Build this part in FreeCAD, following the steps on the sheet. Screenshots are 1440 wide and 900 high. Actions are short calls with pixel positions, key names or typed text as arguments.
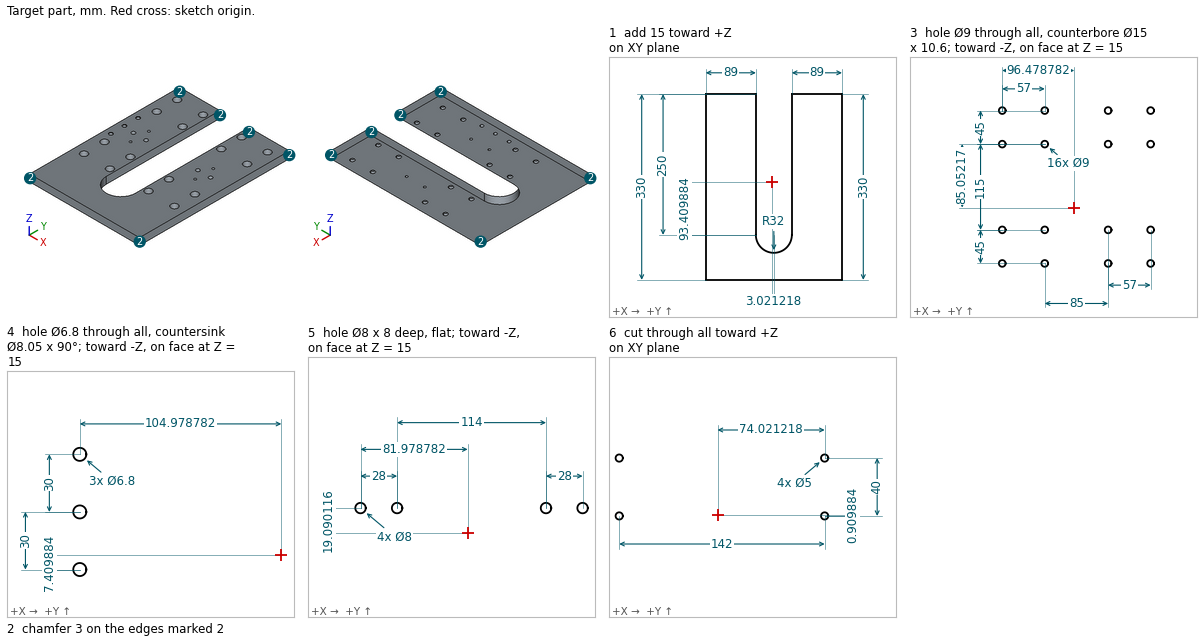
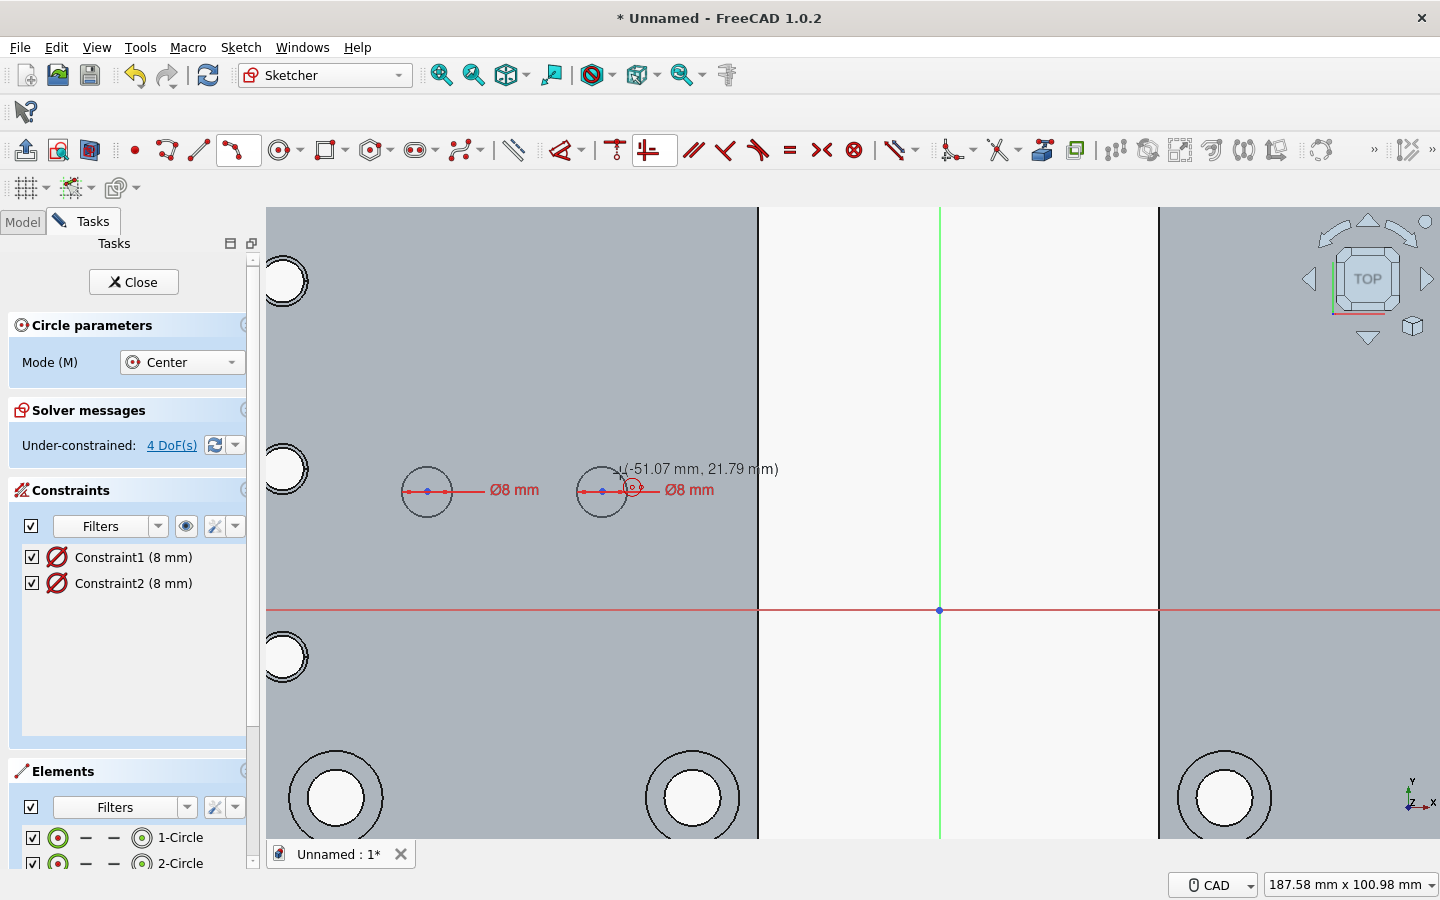
scroll(431, 492, down, 2)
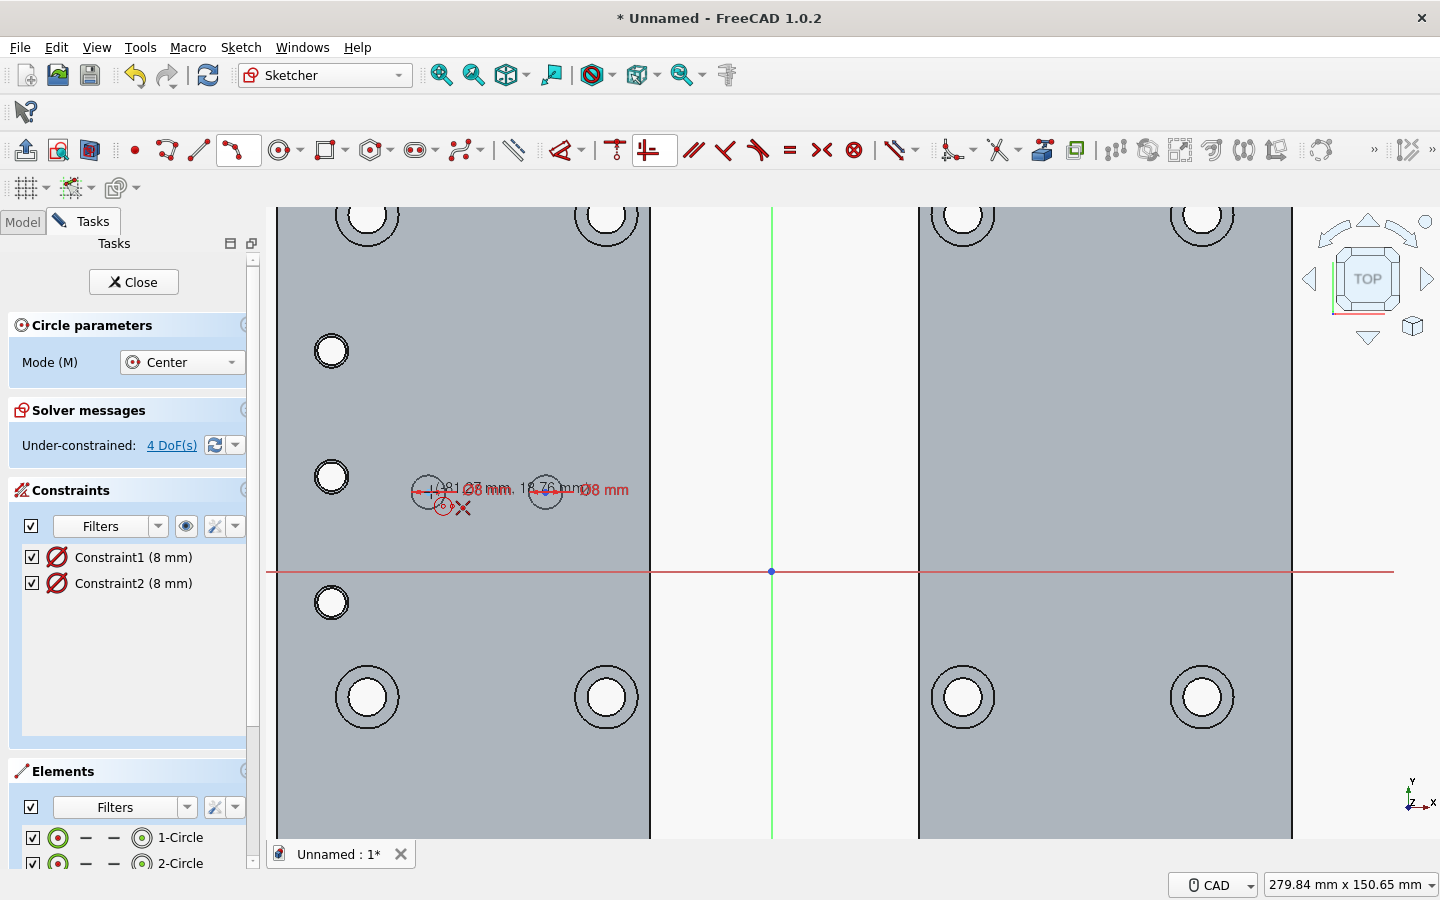
scroll(1024, 491, up, 2)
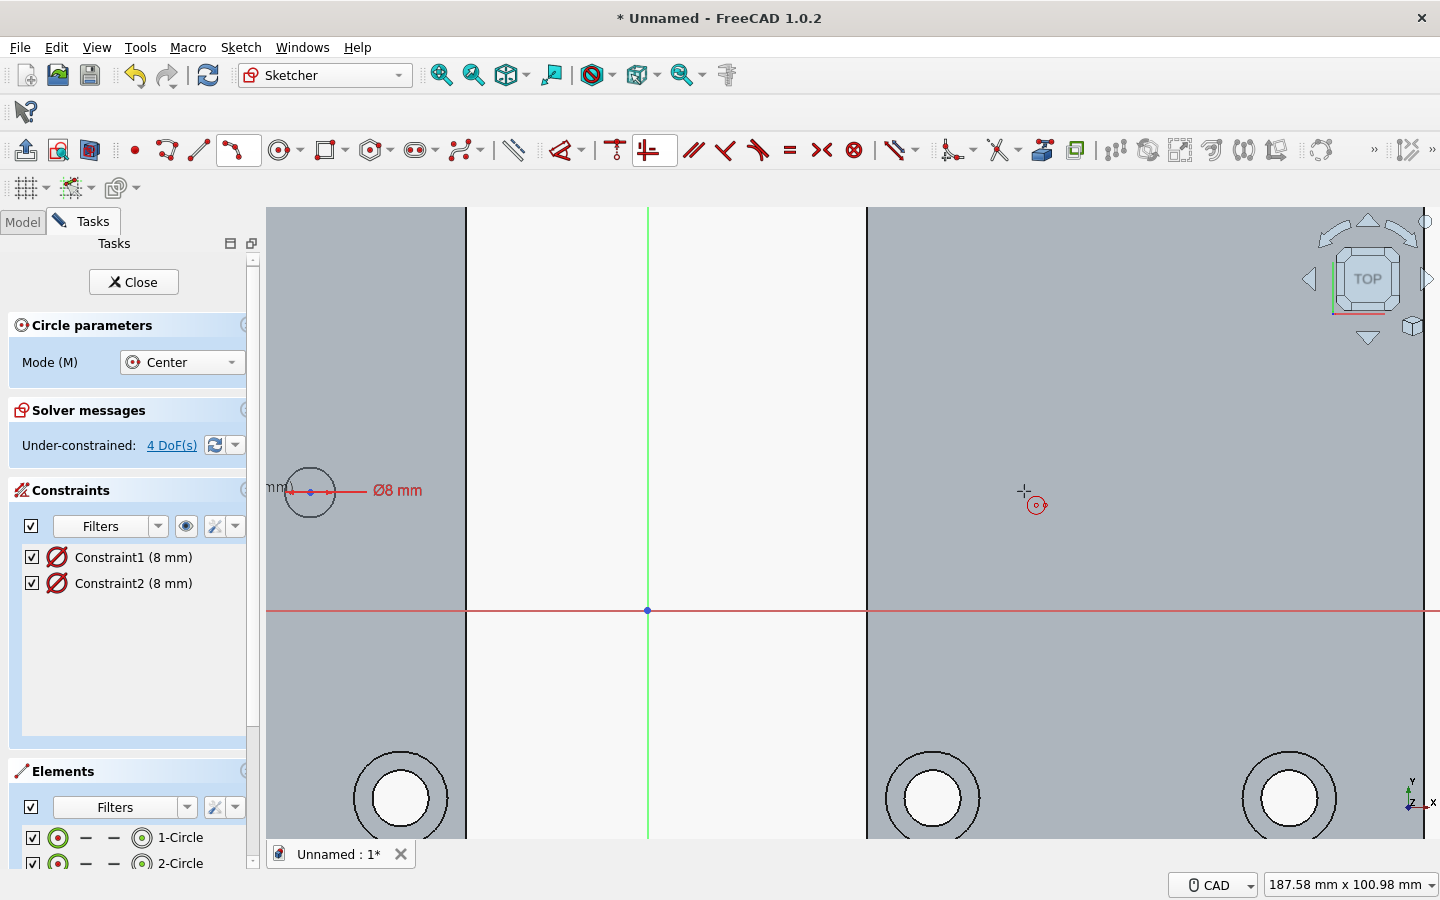
click(1023, 491)
move(1041, 474)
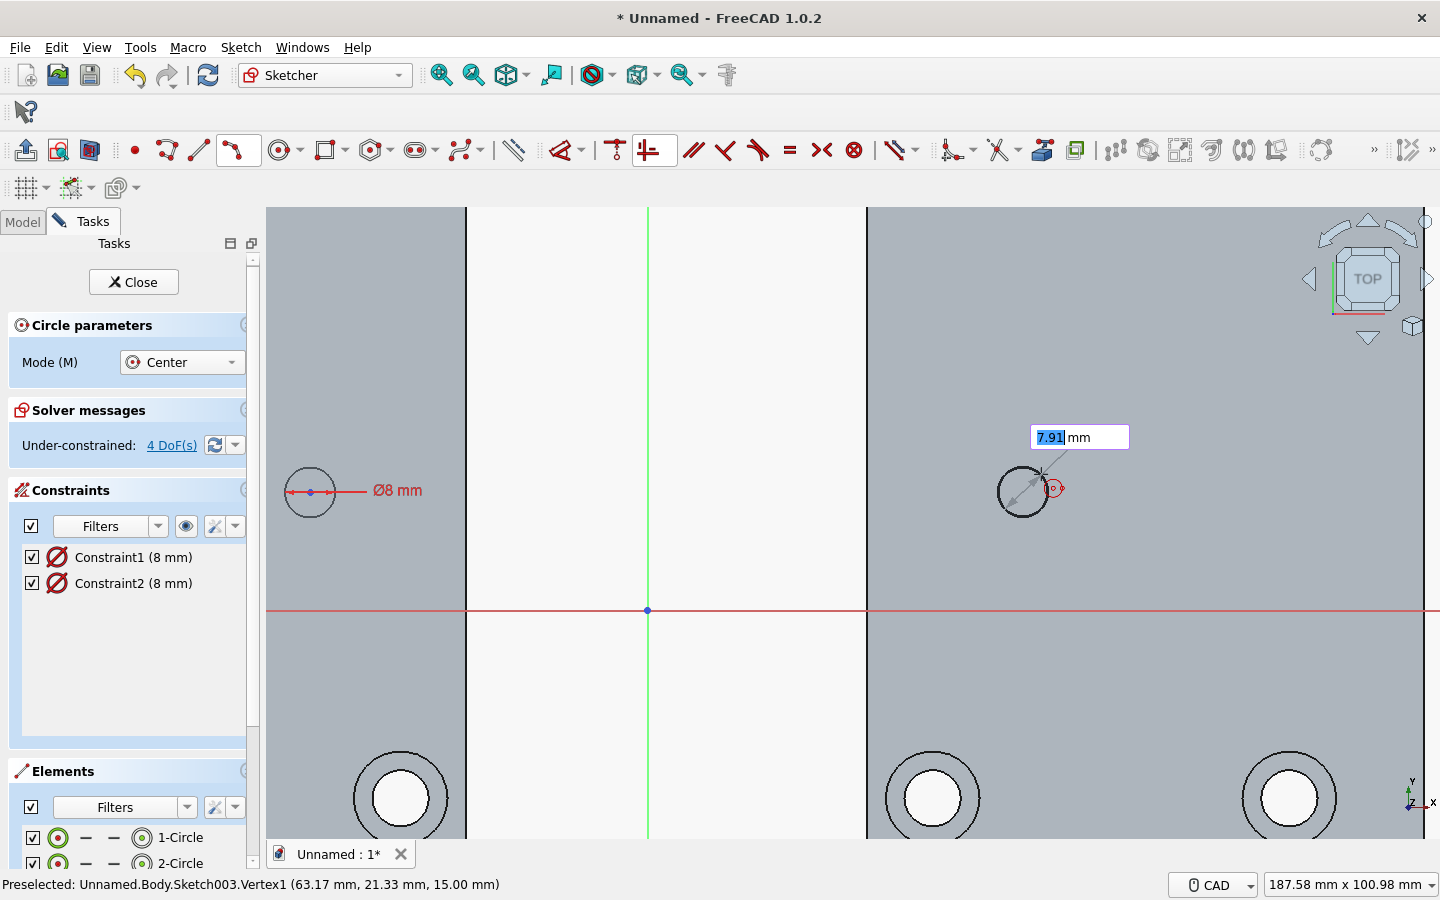
text(8)
key(Return)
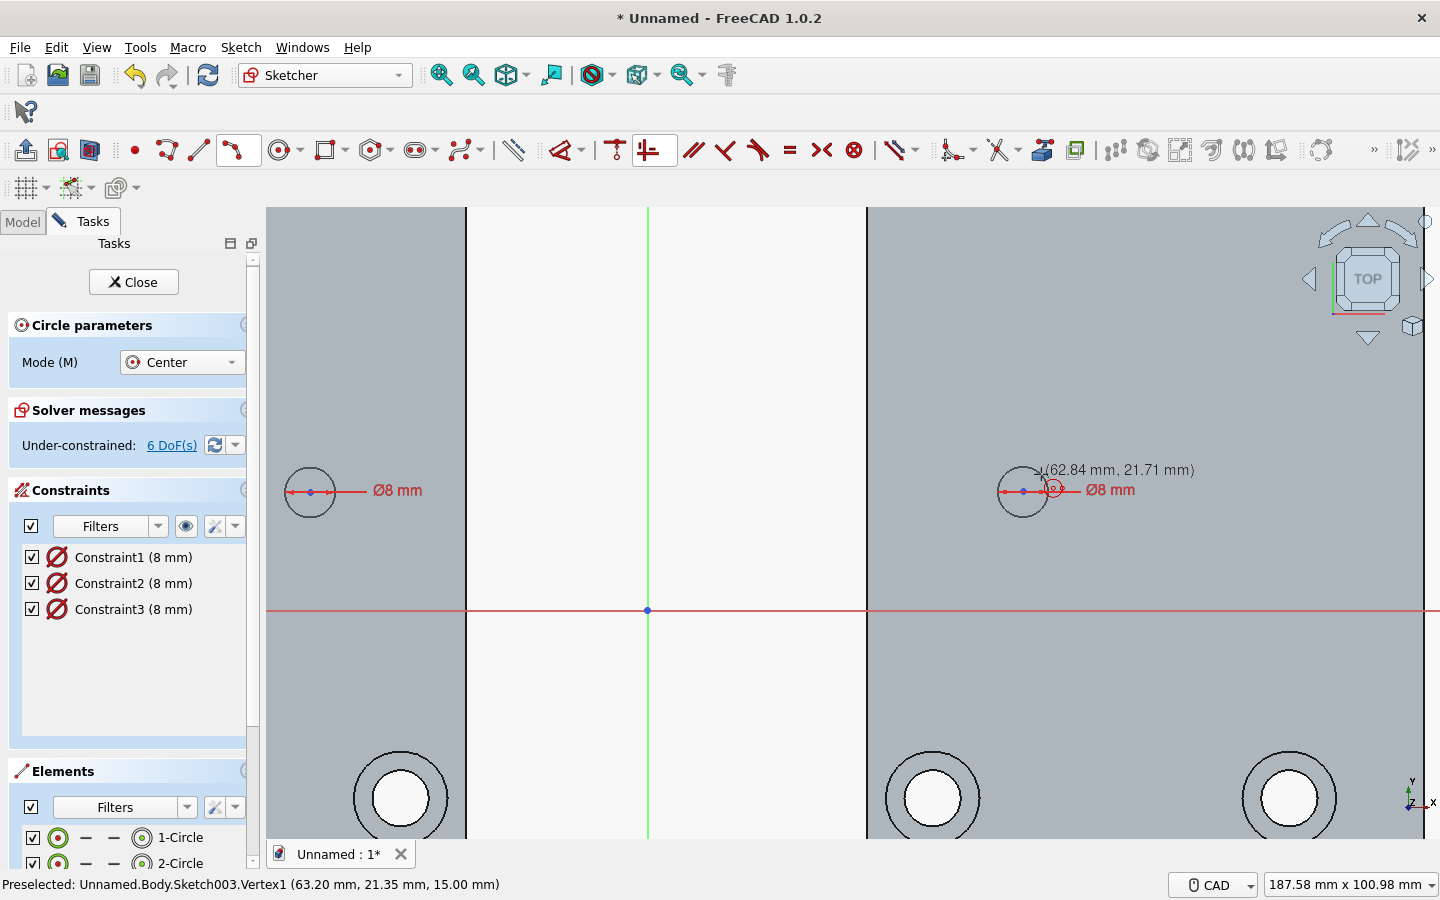
click(1199, 491)
move(1216, 474)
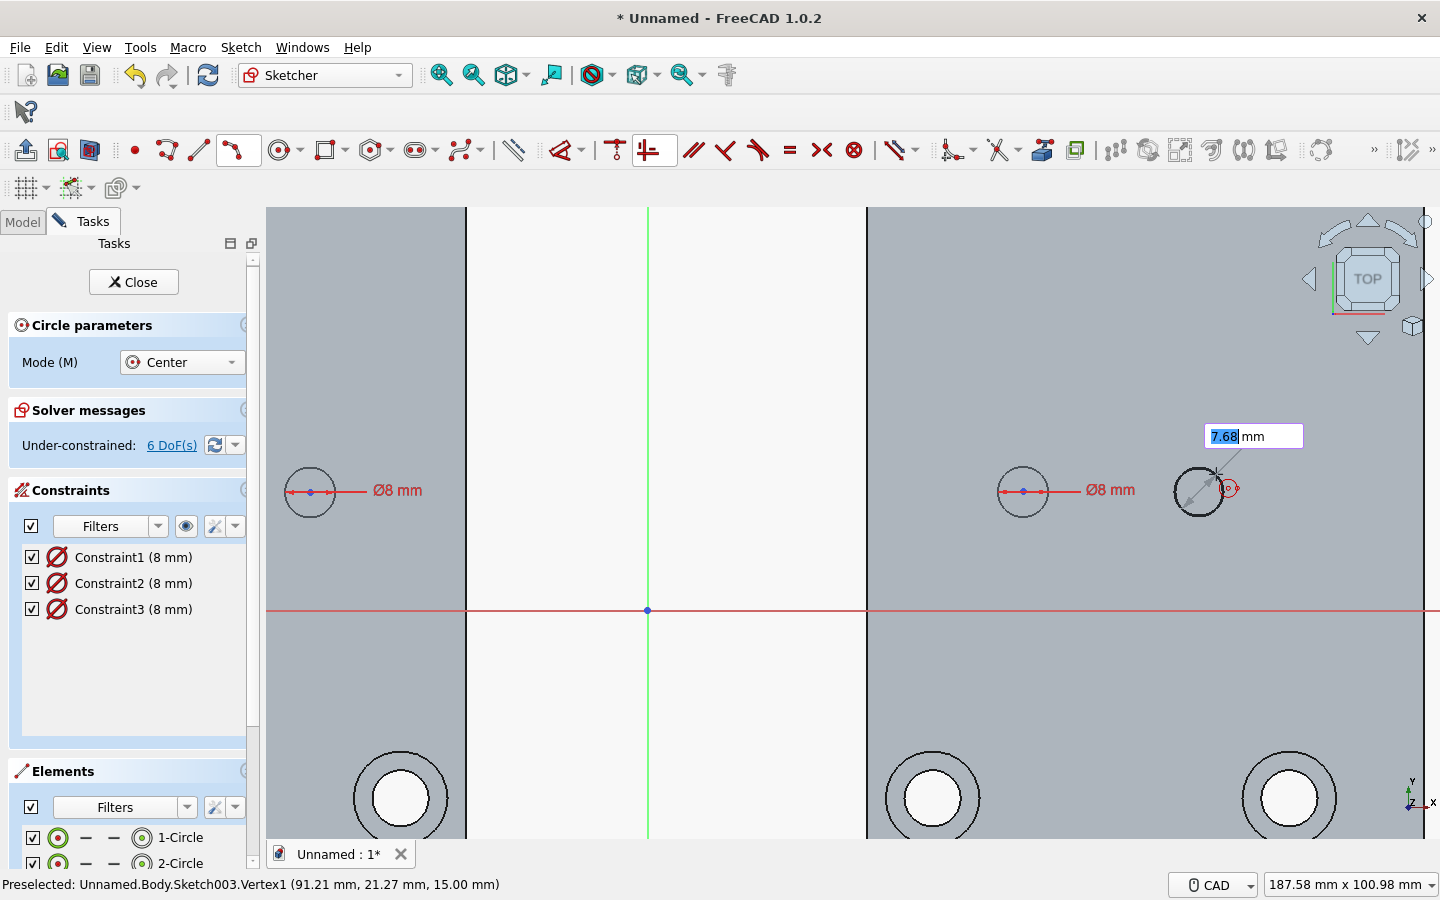
text(8)
key(Return)
key(Escape)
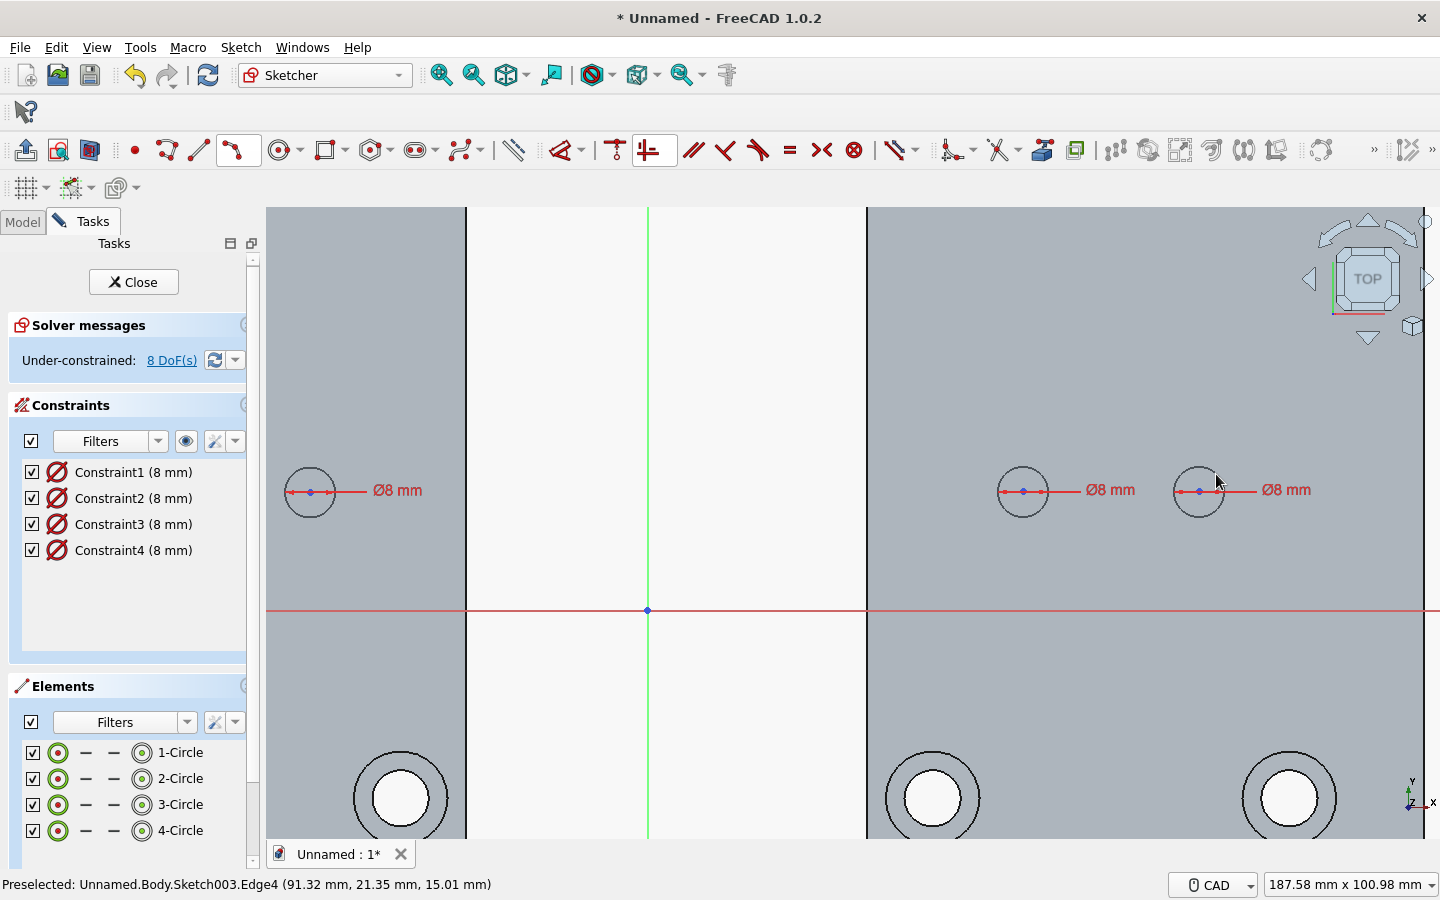
scroll(1024, 491, down, 2)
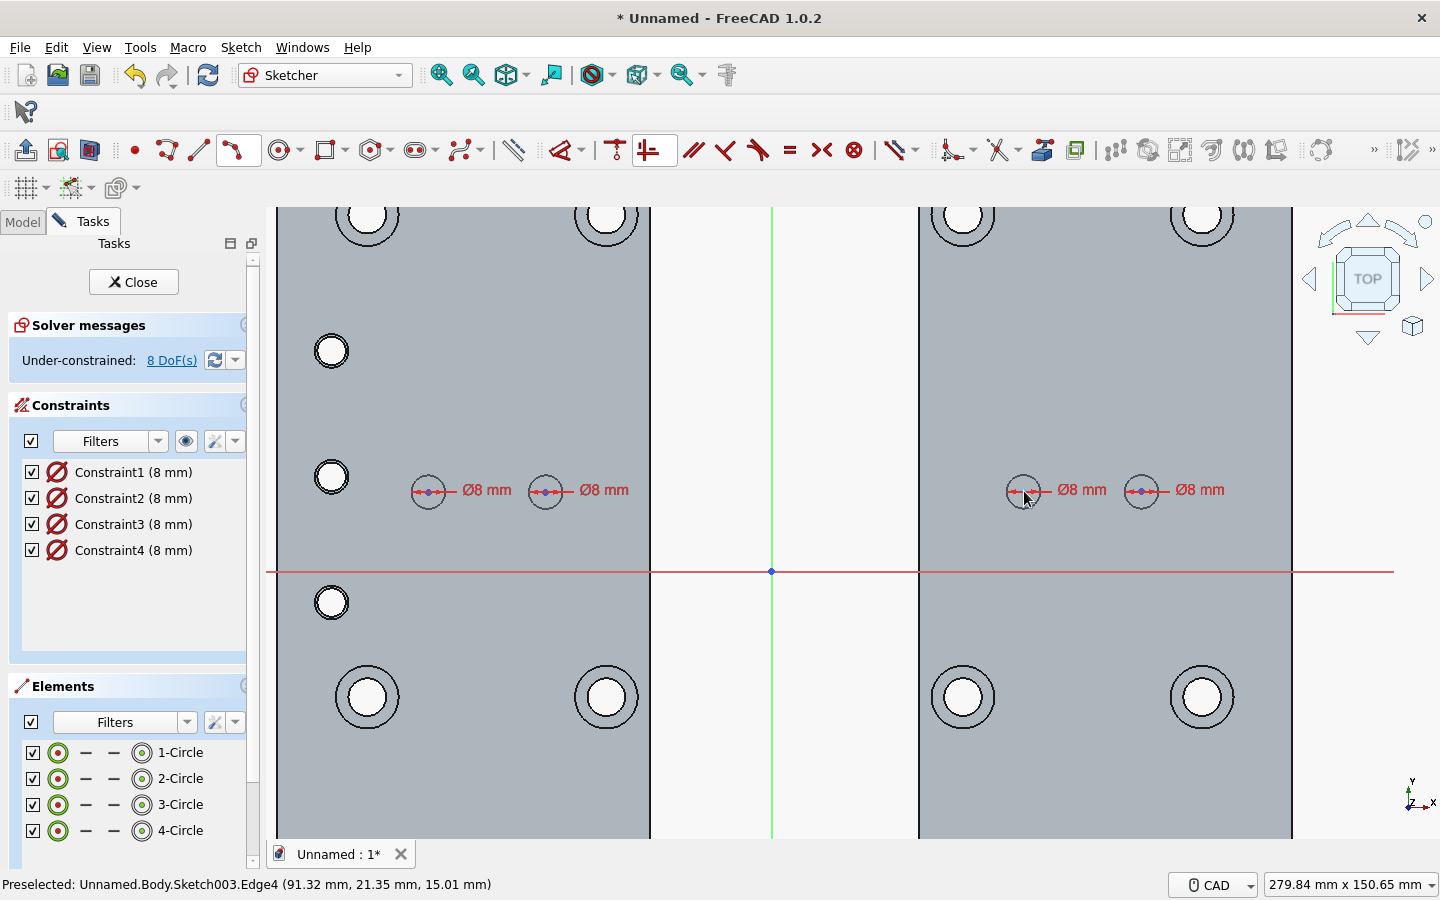
click(428, 492)